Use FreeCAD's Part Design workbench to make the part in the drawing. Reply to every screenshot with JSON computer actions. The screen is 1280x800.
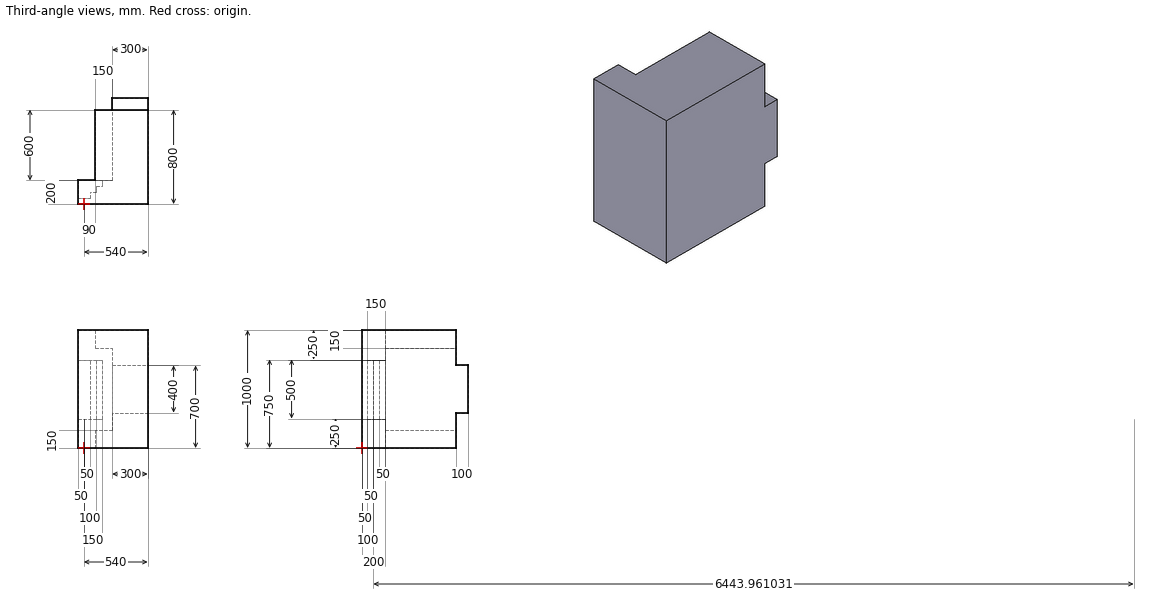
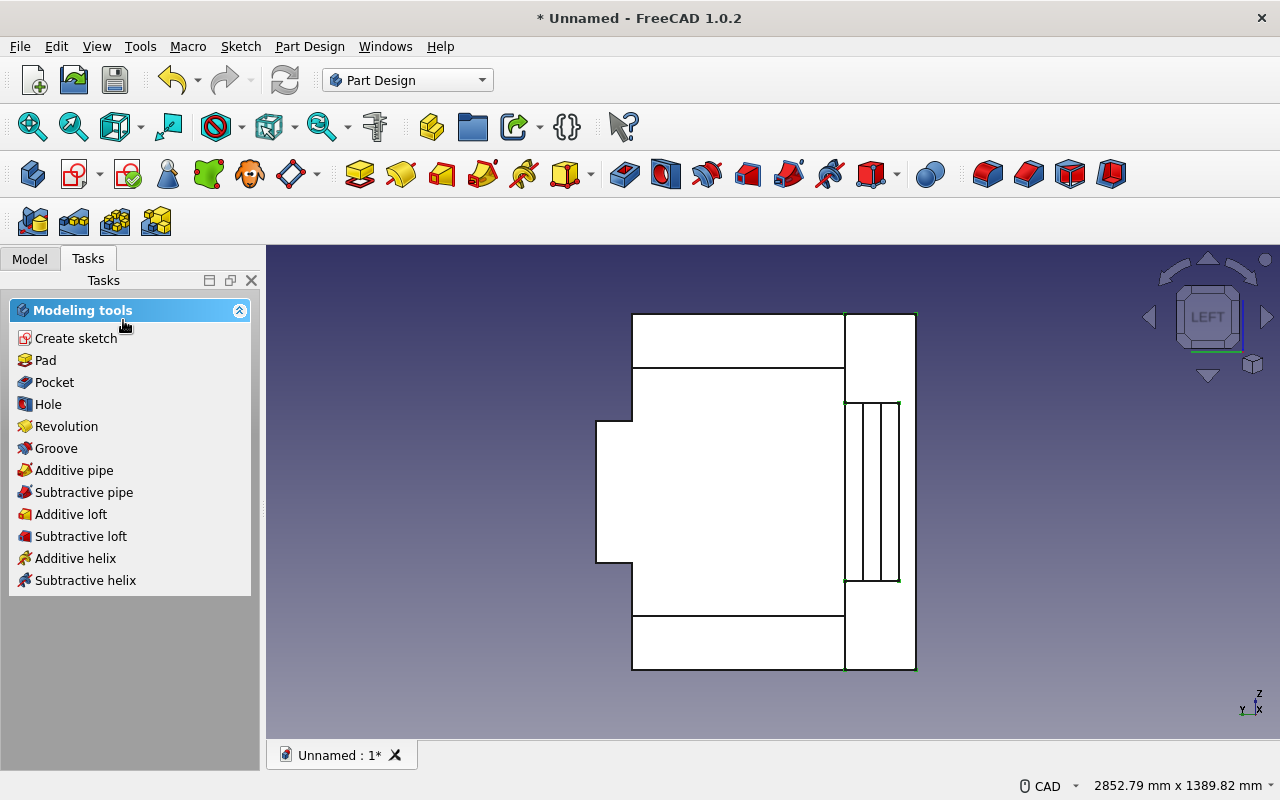
{"action": "left_click", "coordinate": [360, 174]}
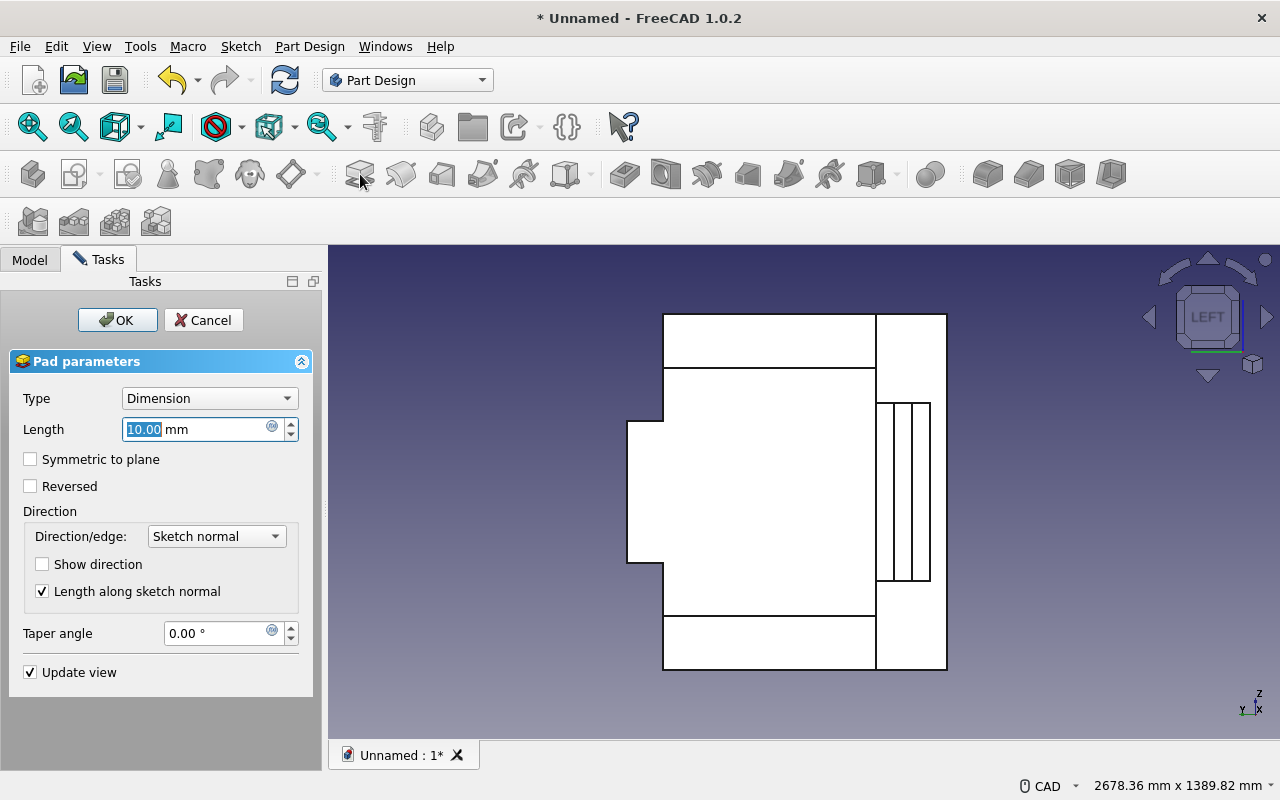
{"action": "type", "text": "50"}
{"action": "key", "text": "Tab"}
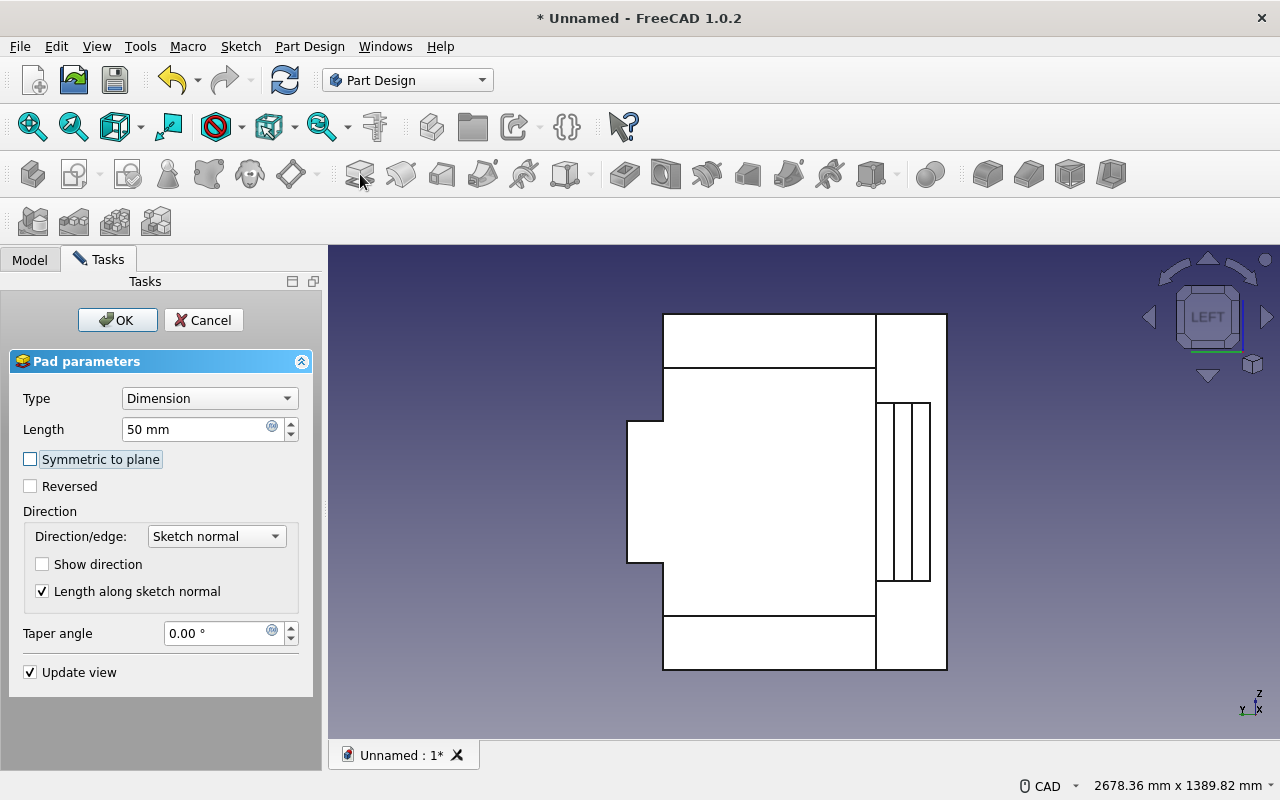
{"action": "left_click", "coordinate": [31, 486]}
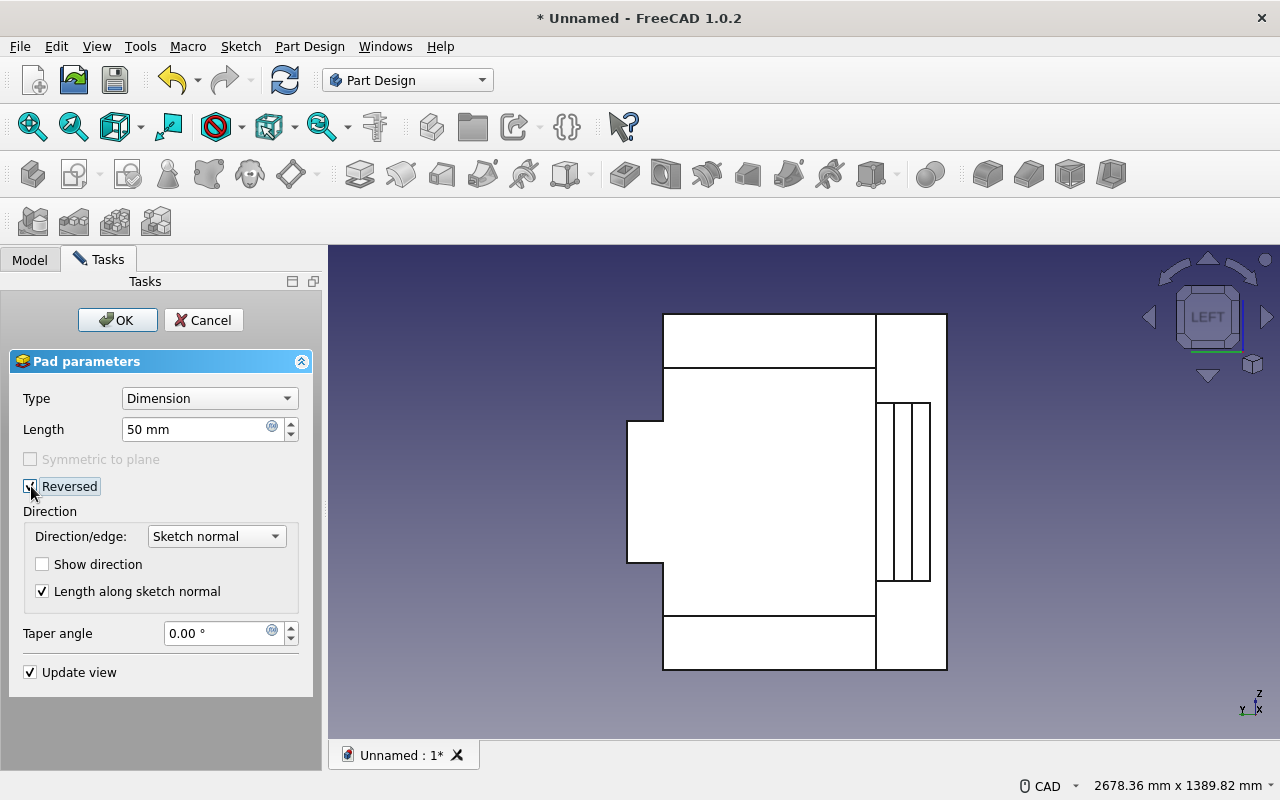
{"action": "left_click", "coordinate": [118, 320]}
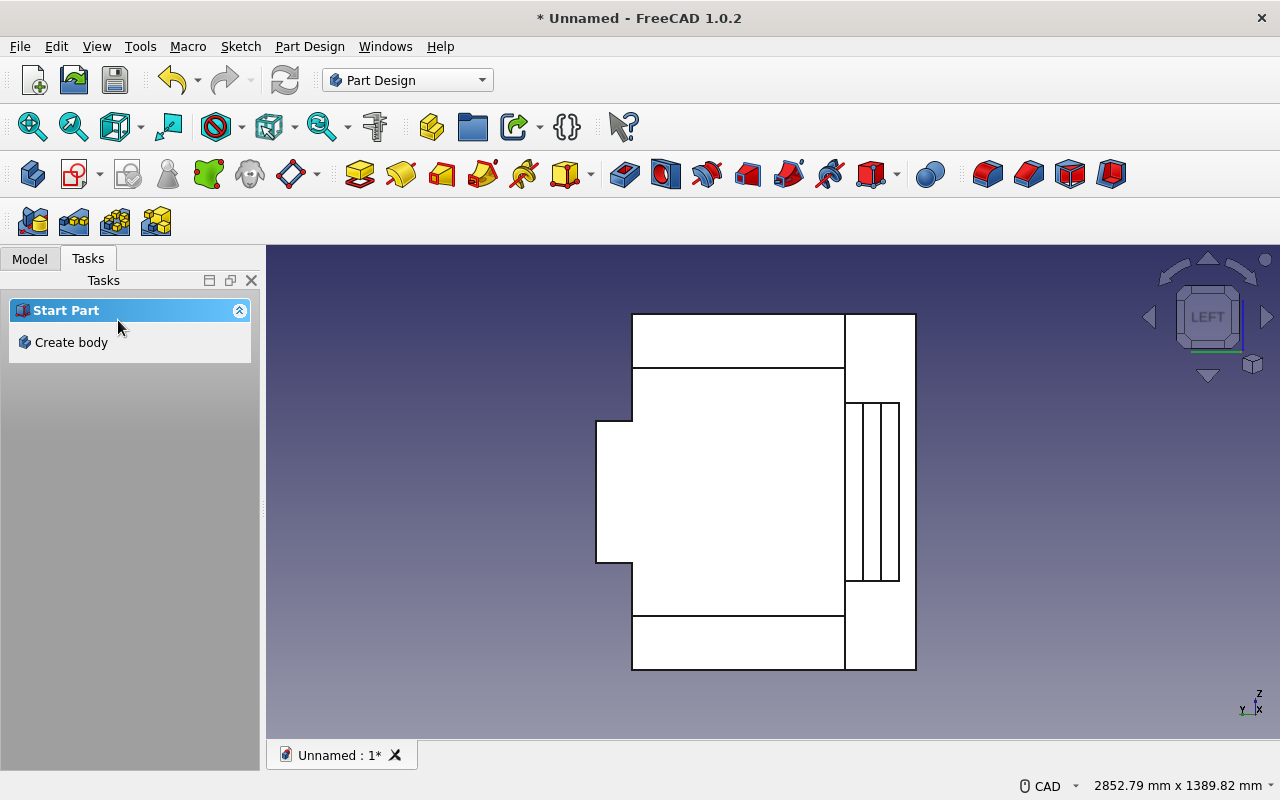
{"action": "key", "text": "0"}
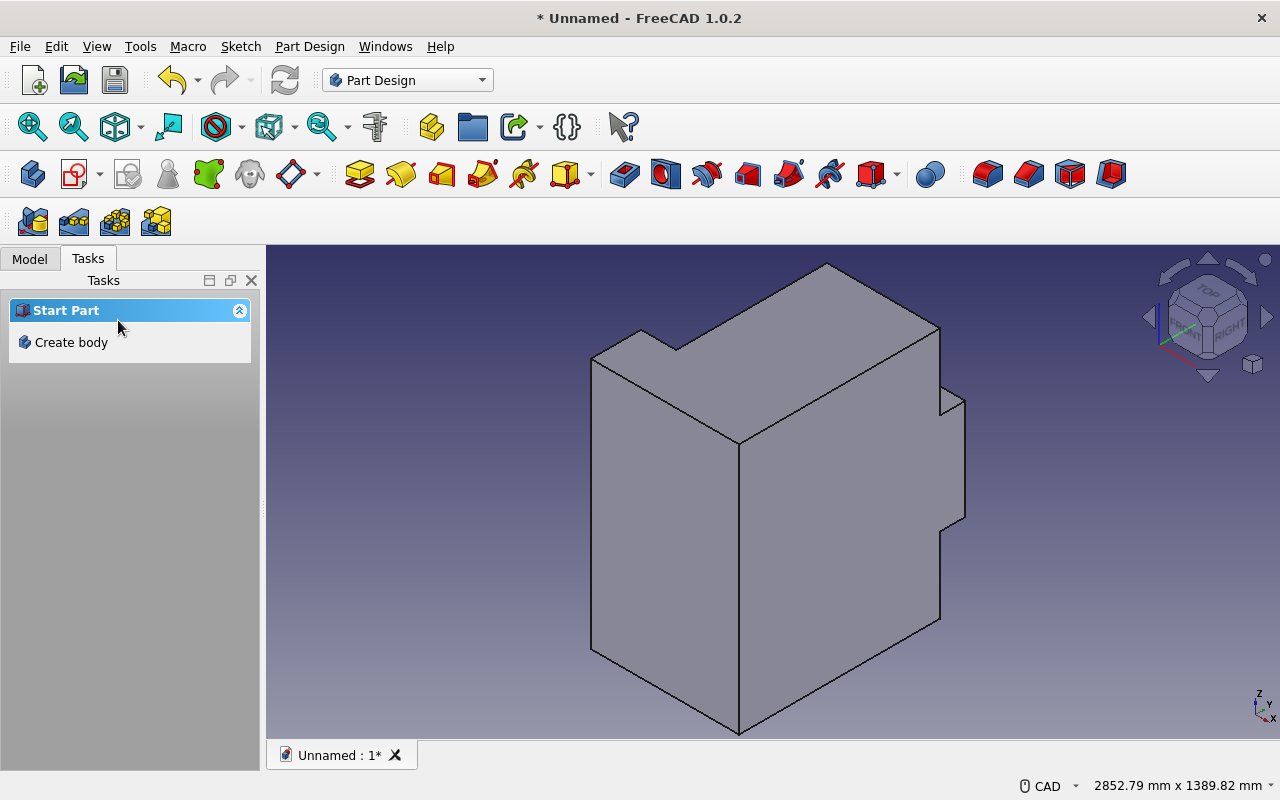
{"action": "left_click", "coordinate": [33, 128]}